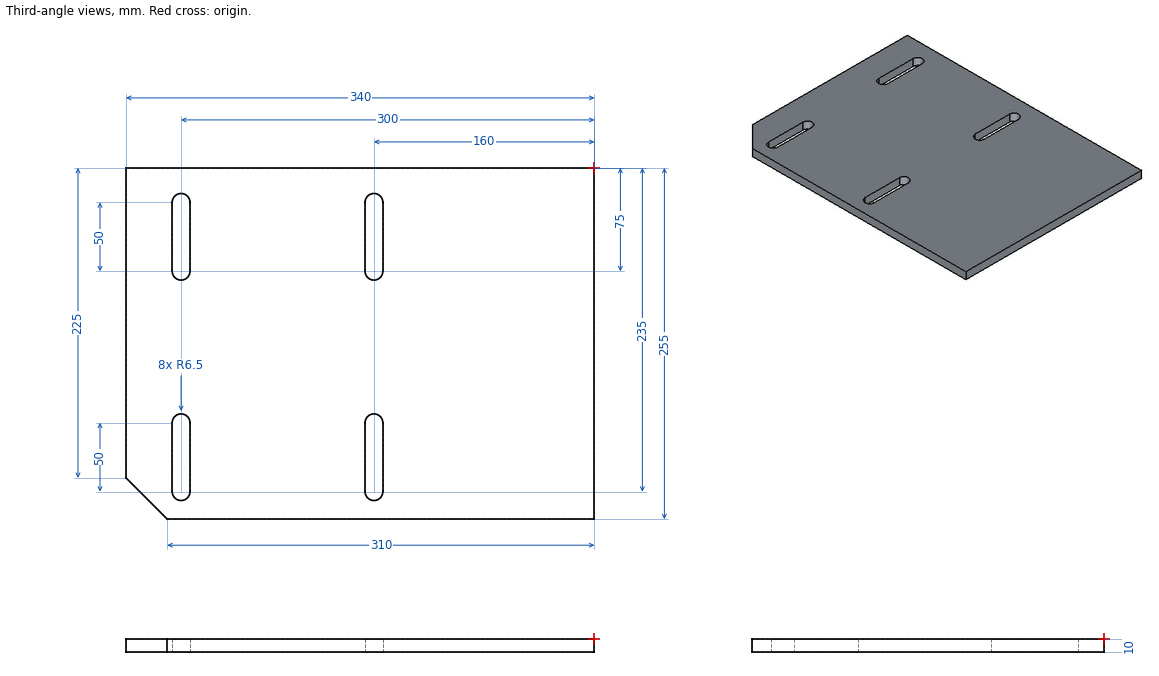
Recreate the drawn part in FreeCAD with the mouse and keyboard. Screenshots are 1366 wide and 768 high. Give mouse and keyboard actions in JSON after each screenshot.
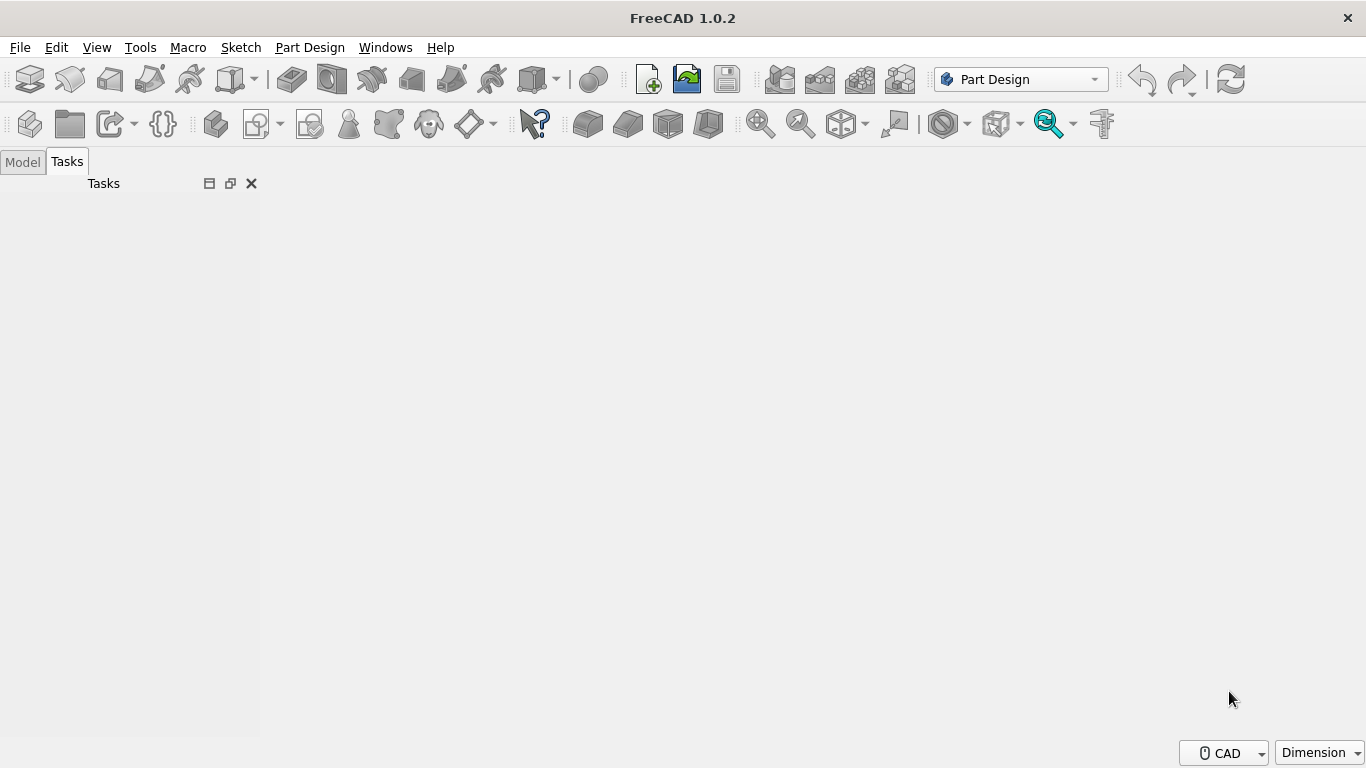
{"action": "key", "text": "ctrl+n"}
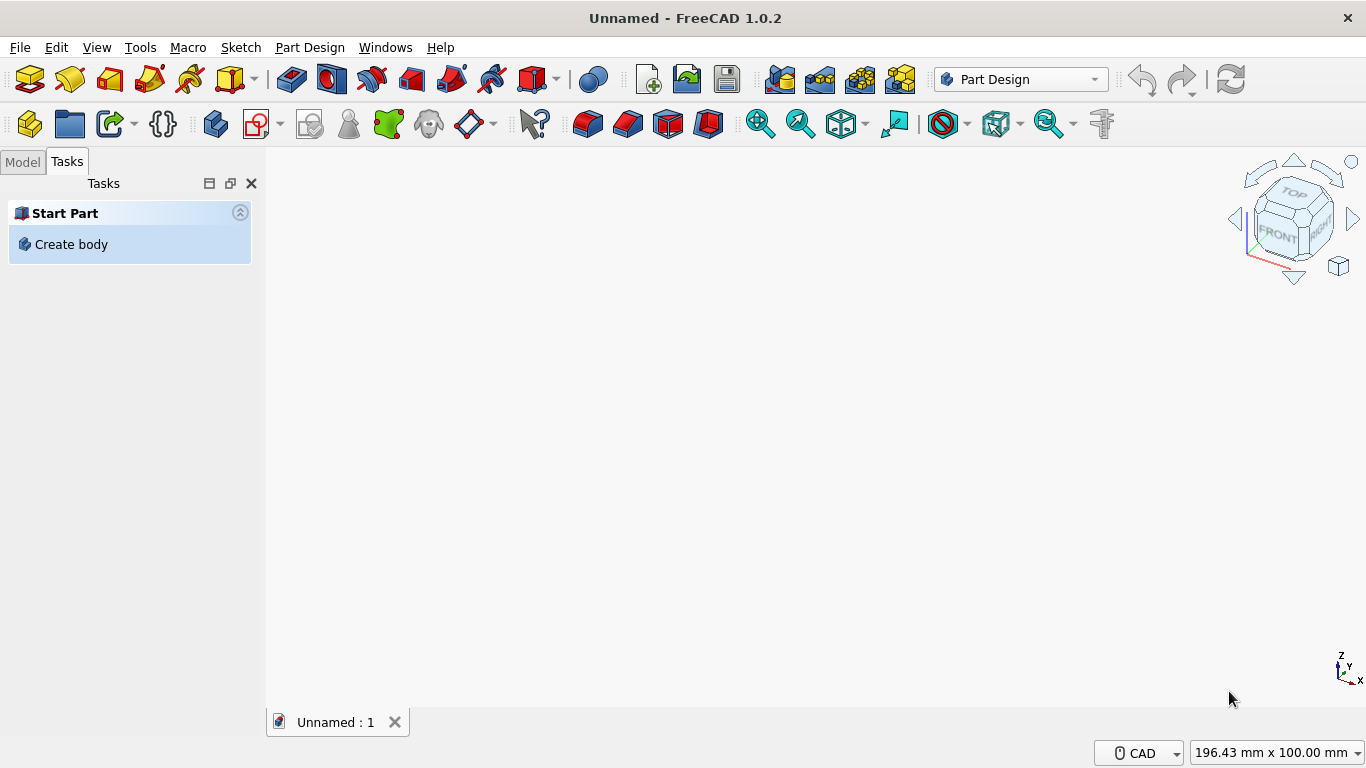
{"action": "left_click", "coordinate": [256, 124]}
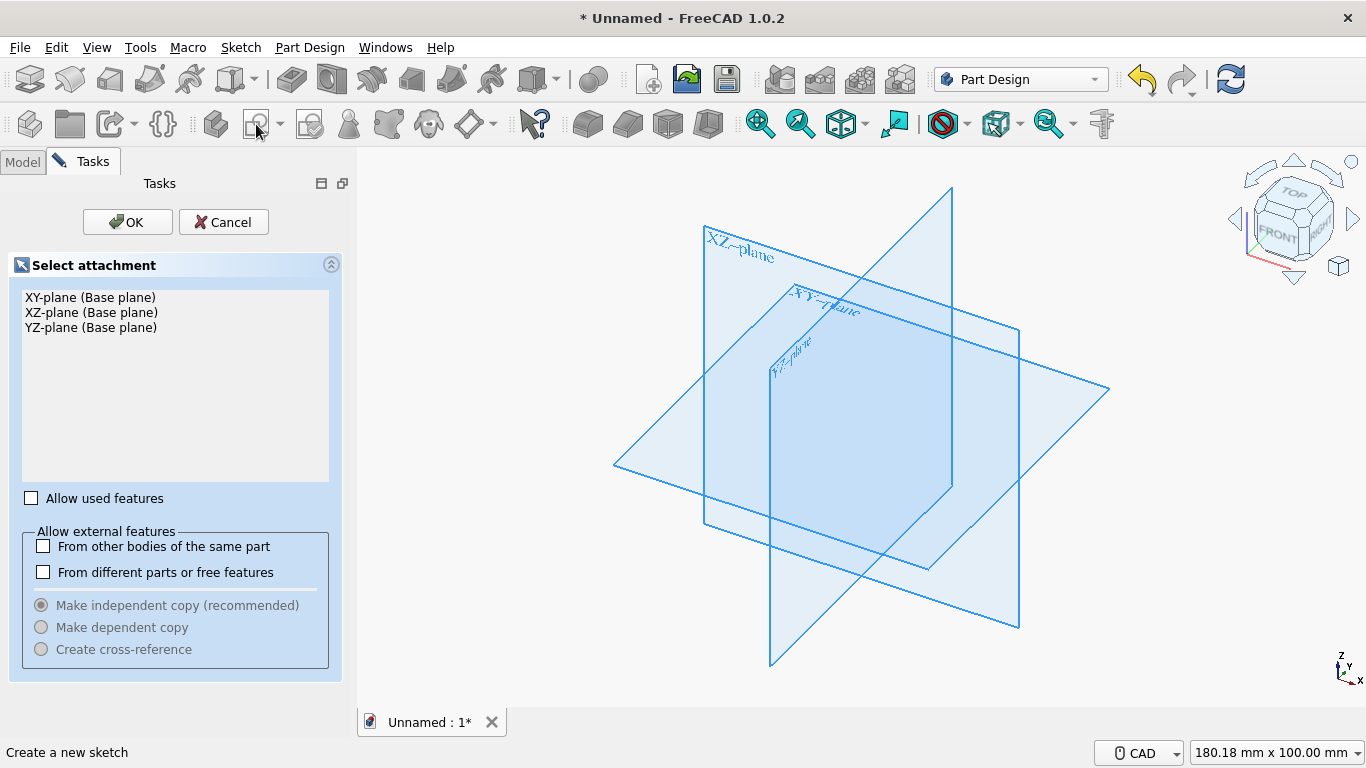
{"action": "left_click", "coordinate": [82, 298]}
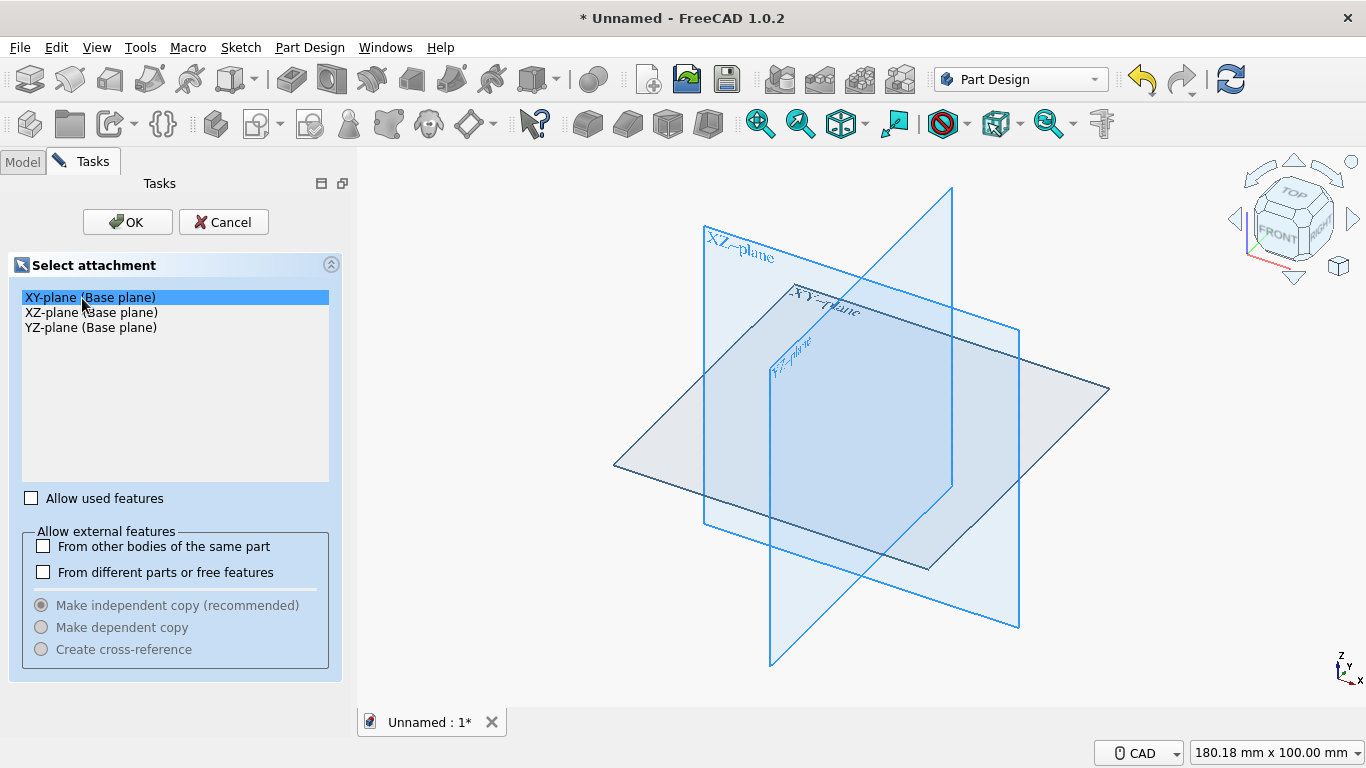
{"action": "left_click", "coordinate": [128, 222]}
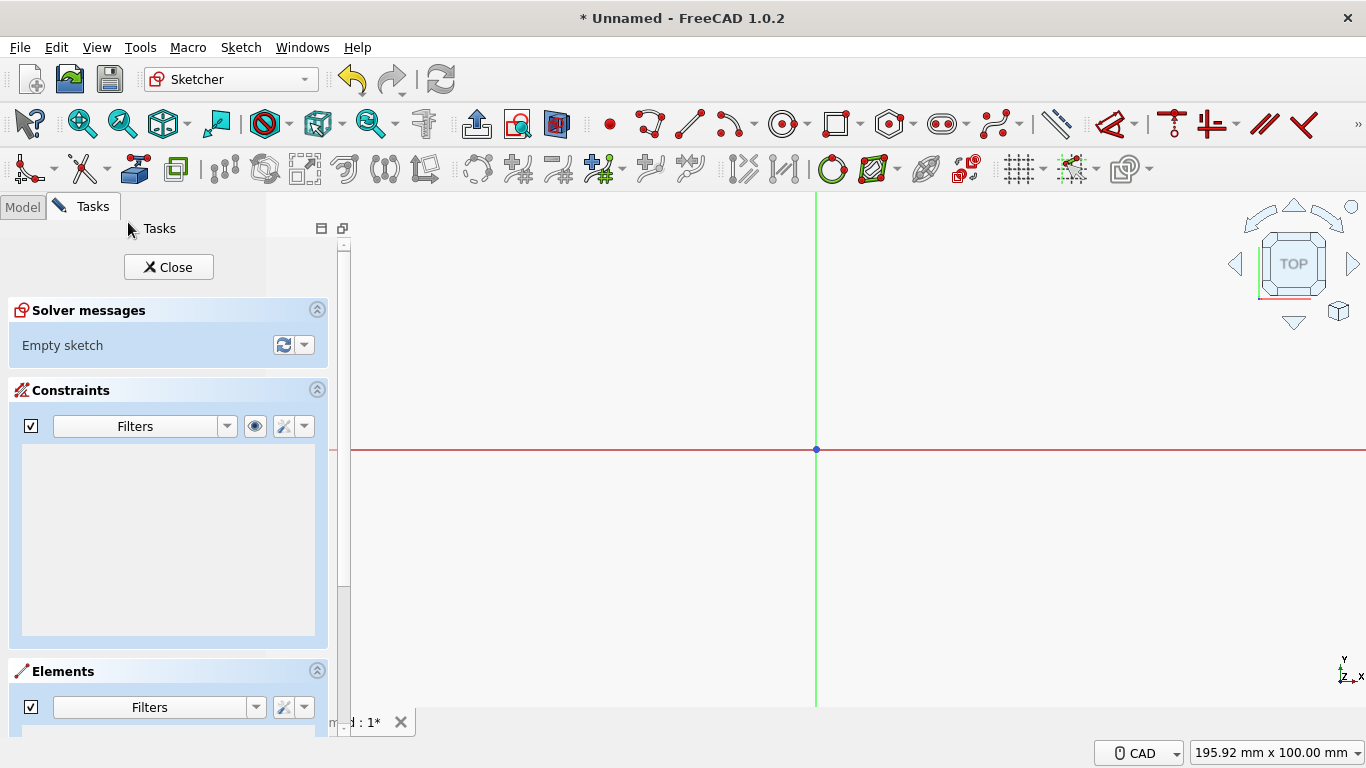
{"action": "scroll", "coordinate": [1012, 235], "scroll_direction": "down", "scroll_amount": 7}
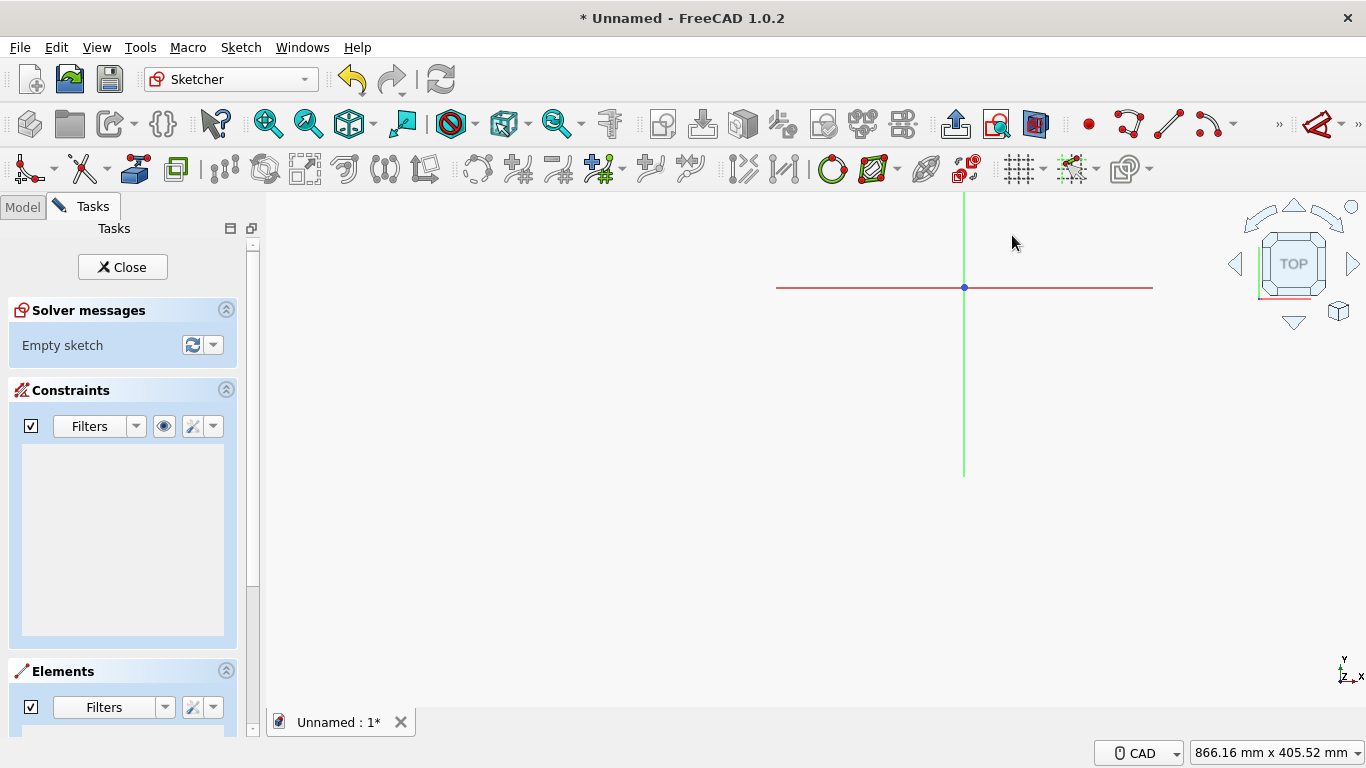
{"action": "key", "text": "g m"}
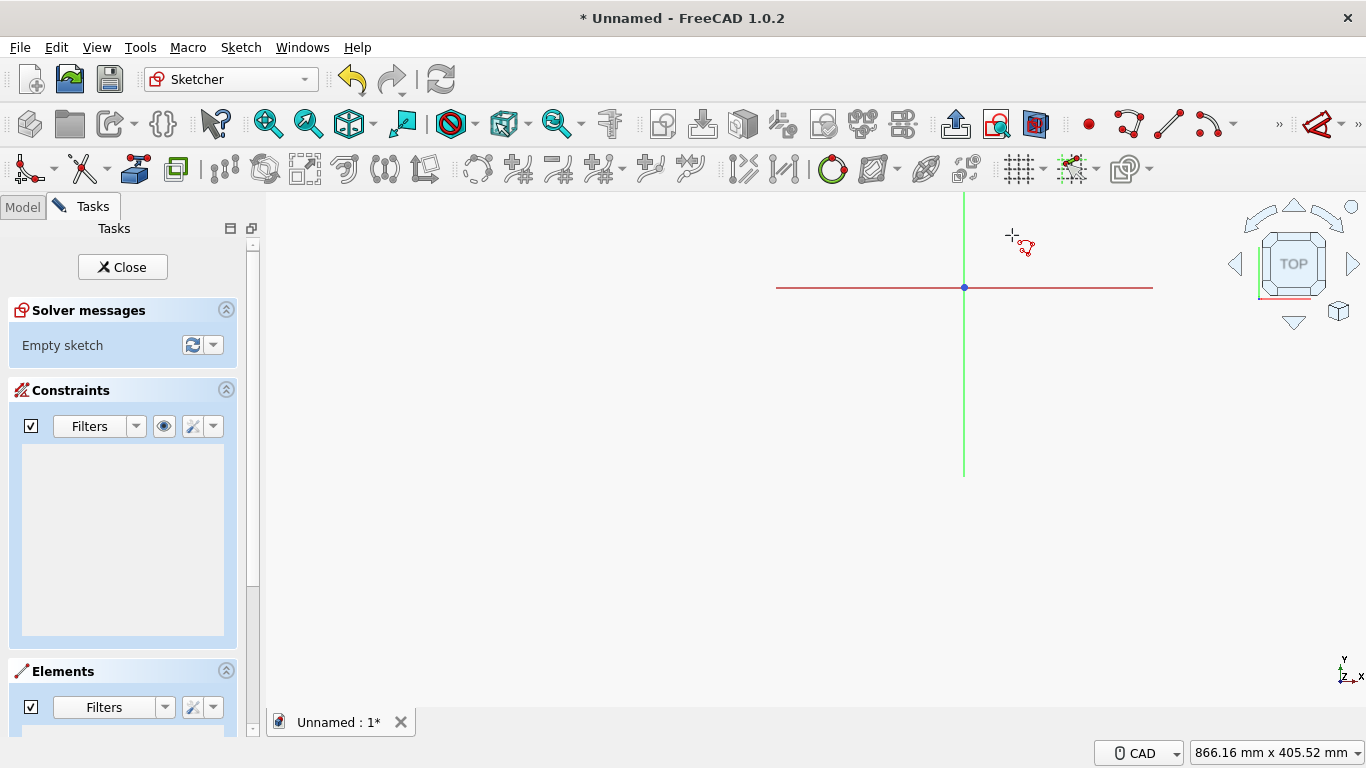
{"action": "left_click", "coordinate": [964, 288]}
{"action": "left_click", "coordinate": [532, 297]}
{"action": "left_click", "coordinate": [532, 574]}
{"action": "left_click", "coordinate": [570, 612]}
{"action": "left_click", "coordinate": [955, 612]}
{"action": "left_click", "coordinate": [964, 288]}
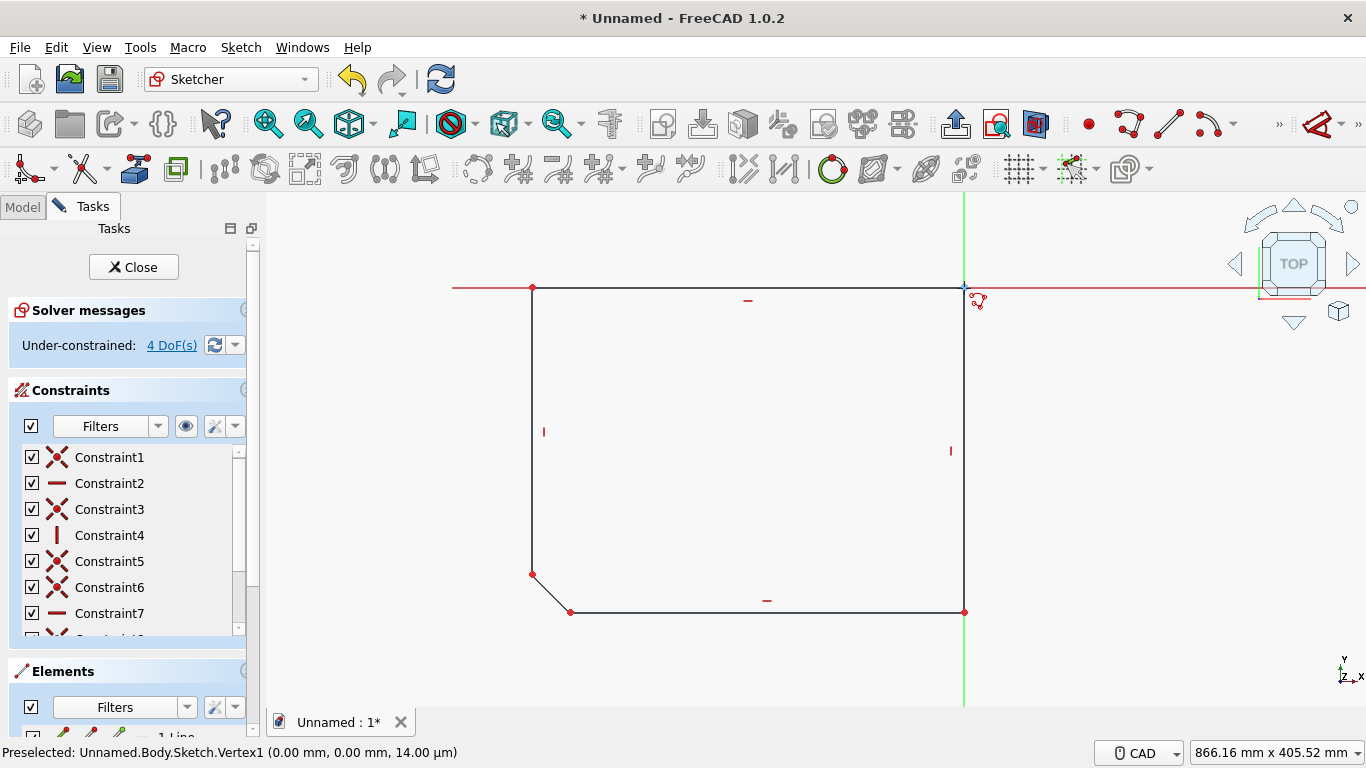
{"action": "key", "text": "g s"}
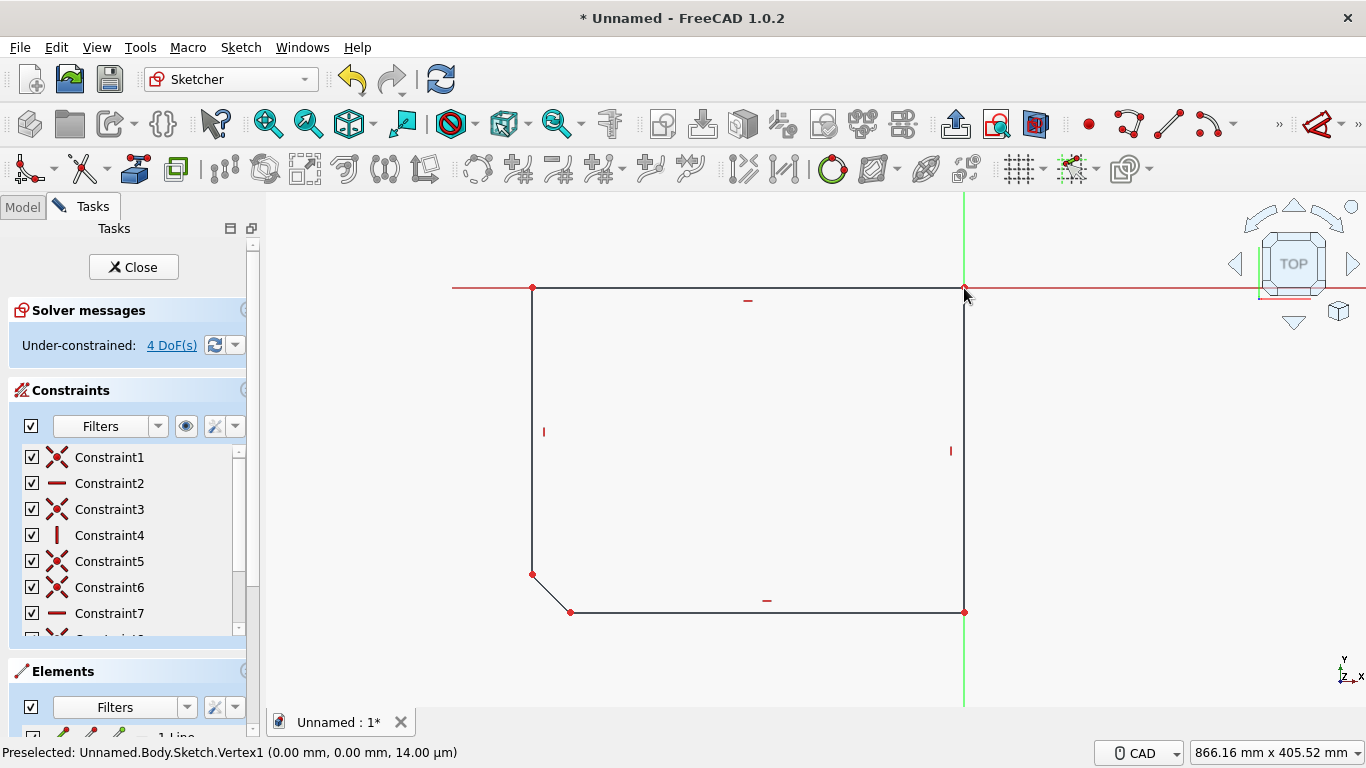
{"action": "scroll", "coordinate": [583, 586], "scroll_direction": "up", "scroll_amount": 6}